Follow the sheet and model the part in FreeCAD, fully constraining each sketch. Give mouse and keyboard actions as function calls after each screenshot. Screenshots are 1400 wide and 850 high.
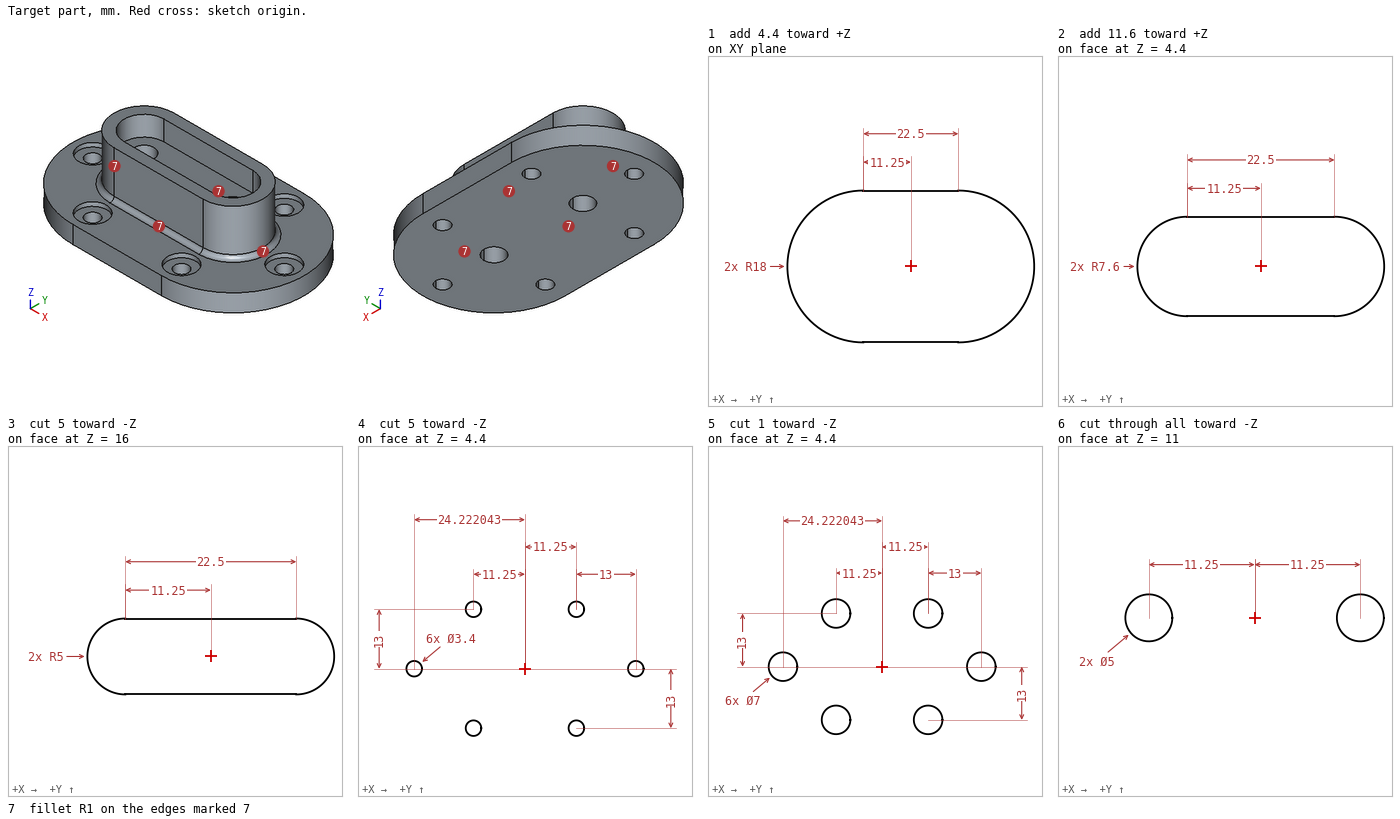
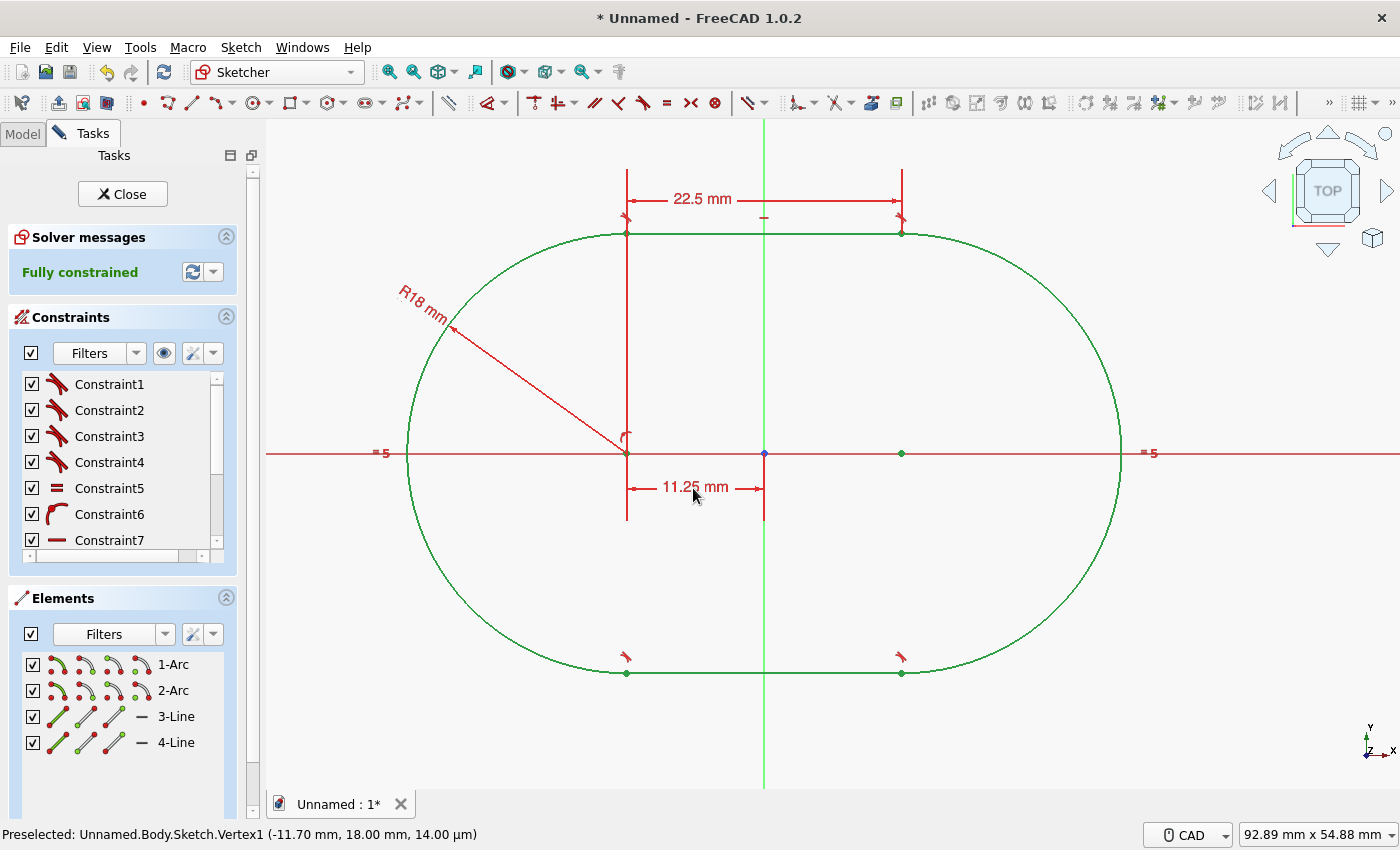
click(123, 194)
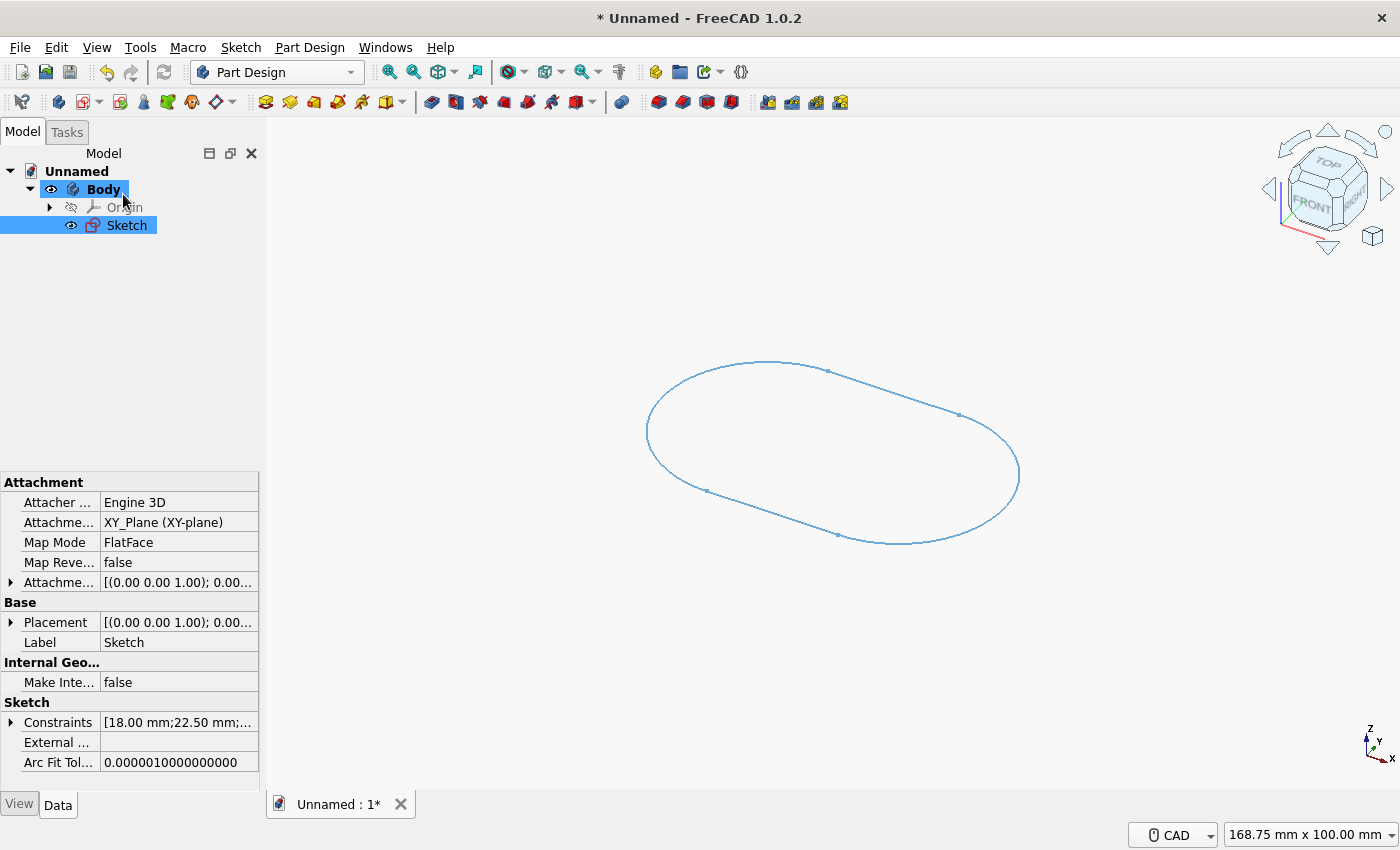
click(266, 102)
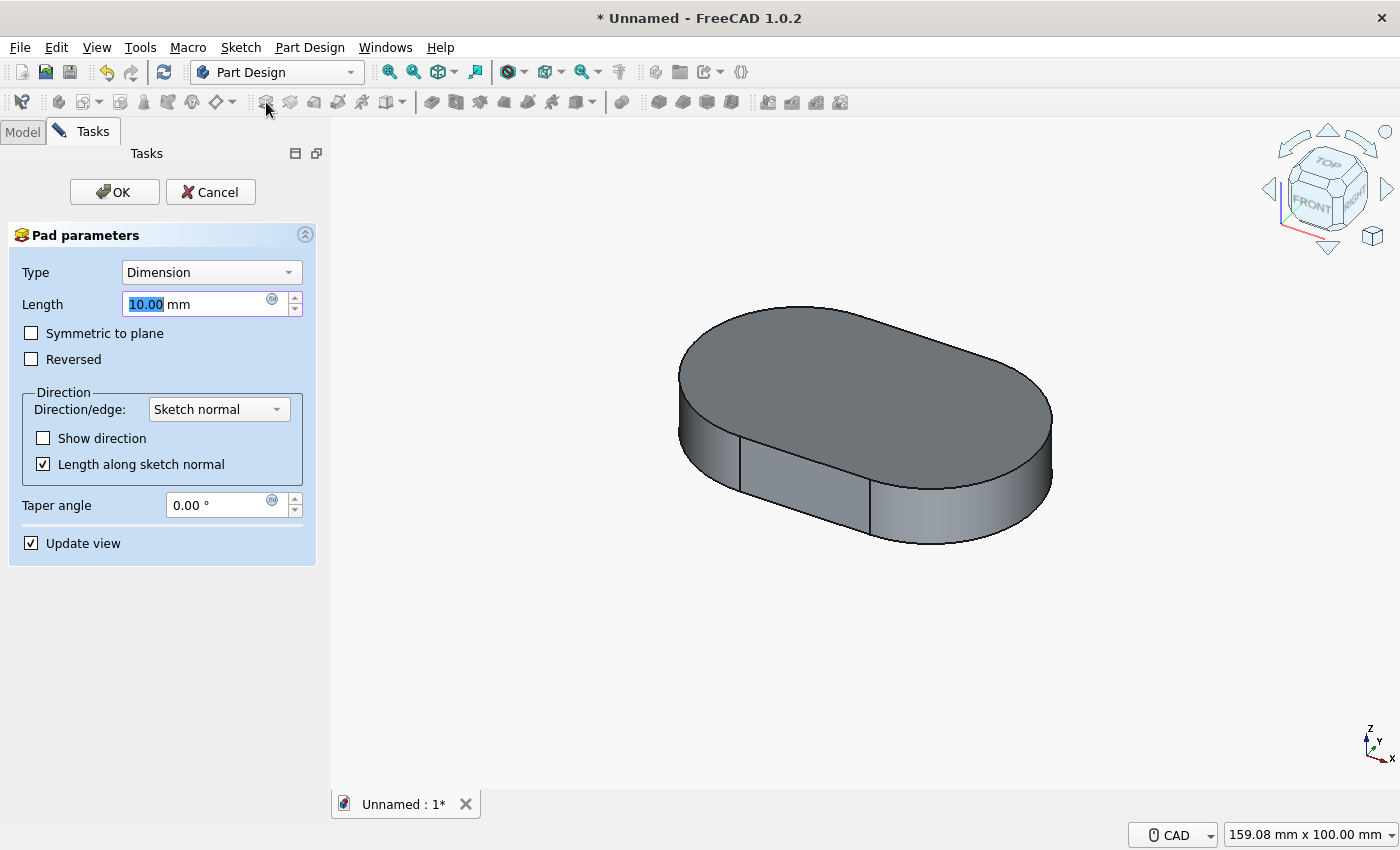
text(4.4)
key(Tab)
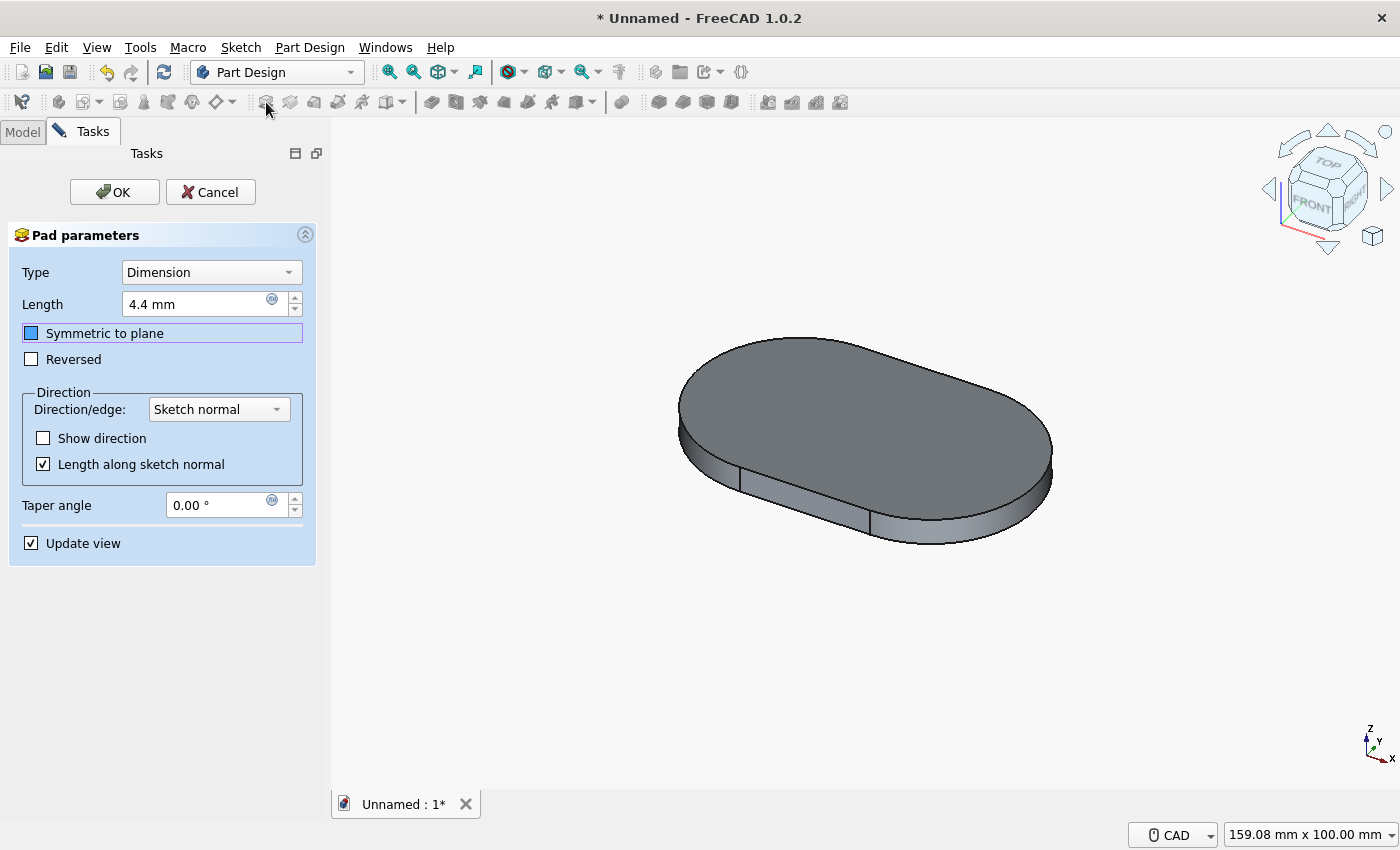
click(115, 192)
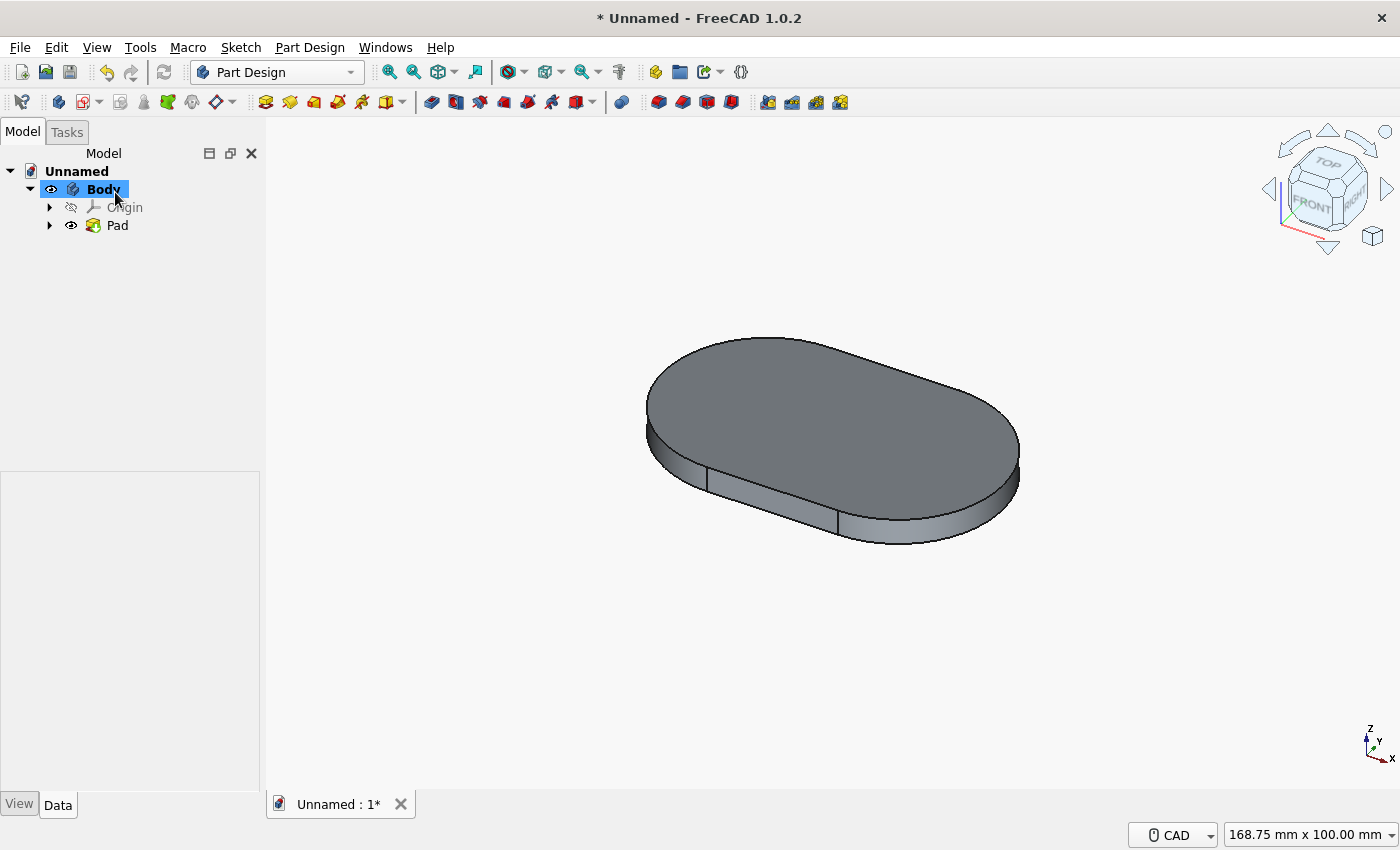
click(390, 72)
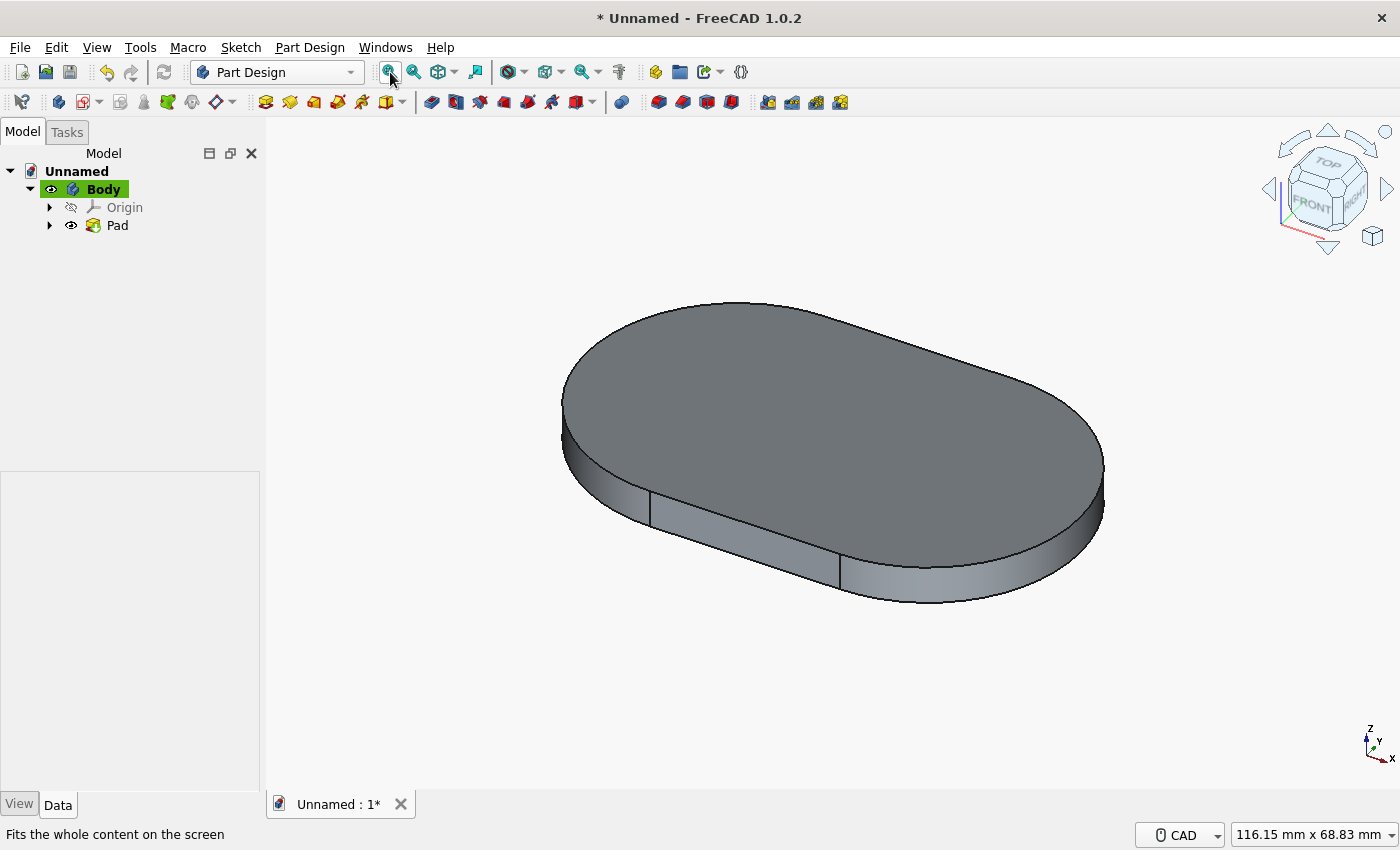
click(904, 458)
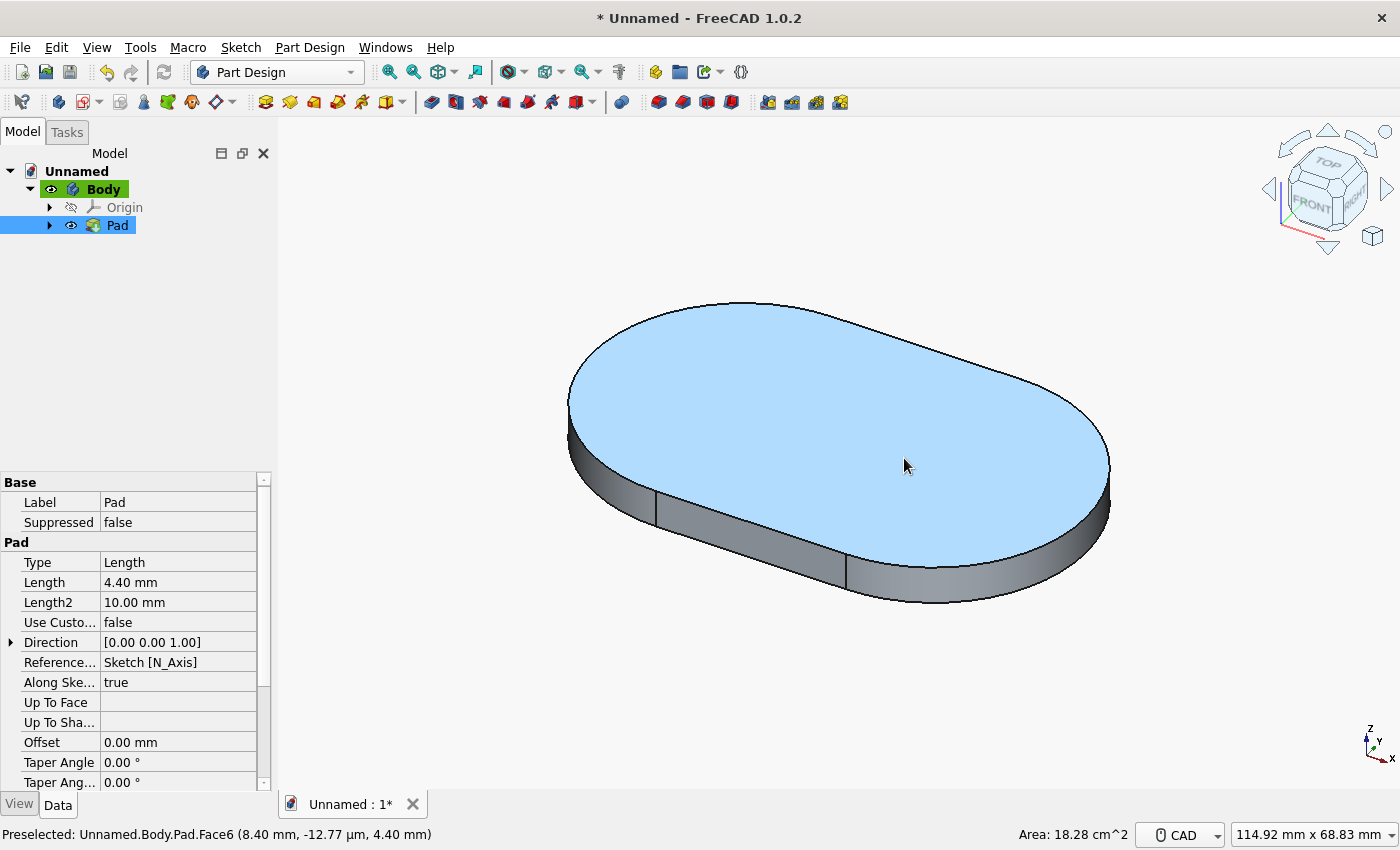
click(84, 102)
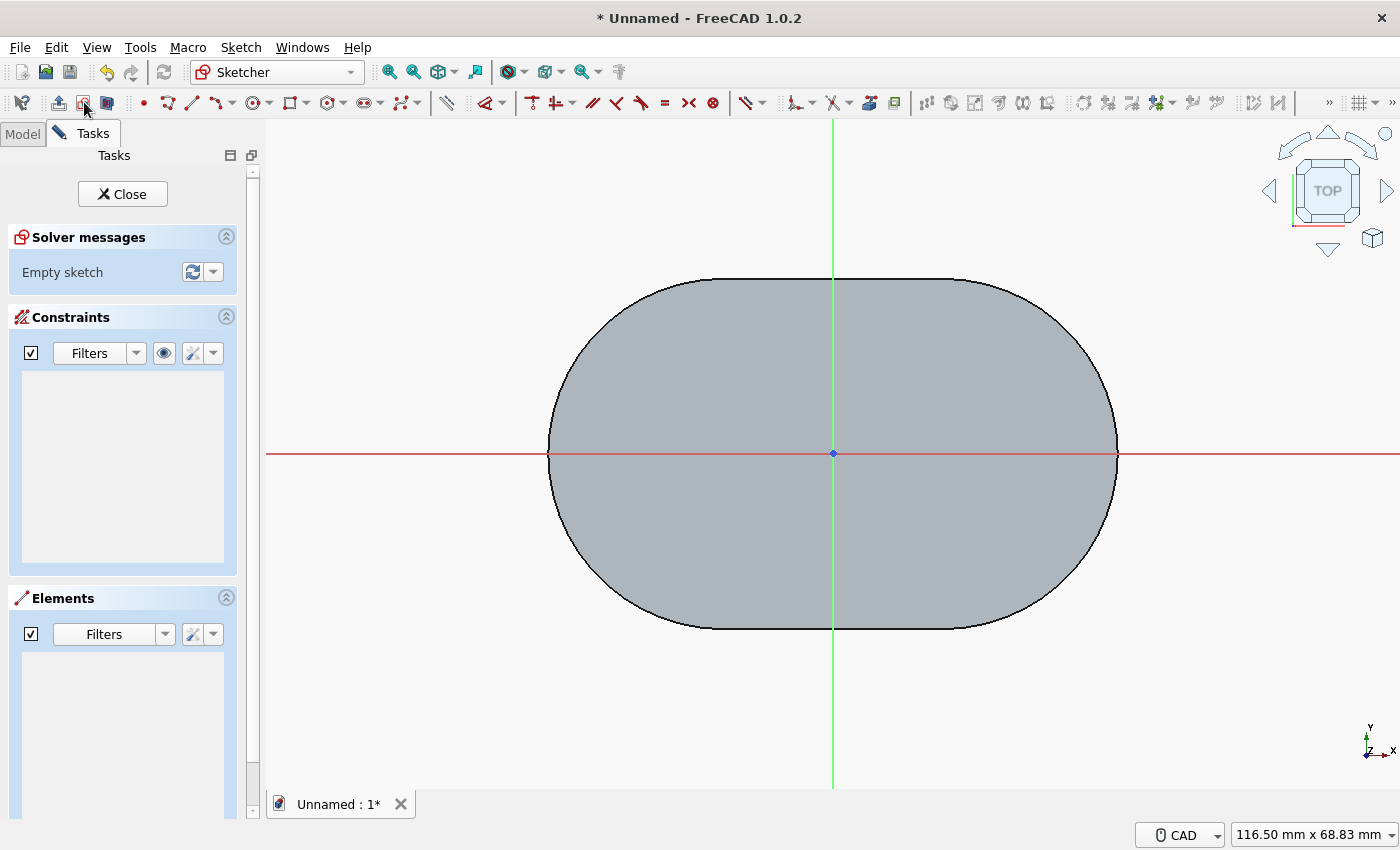
scroll(916, 454, up, 3)